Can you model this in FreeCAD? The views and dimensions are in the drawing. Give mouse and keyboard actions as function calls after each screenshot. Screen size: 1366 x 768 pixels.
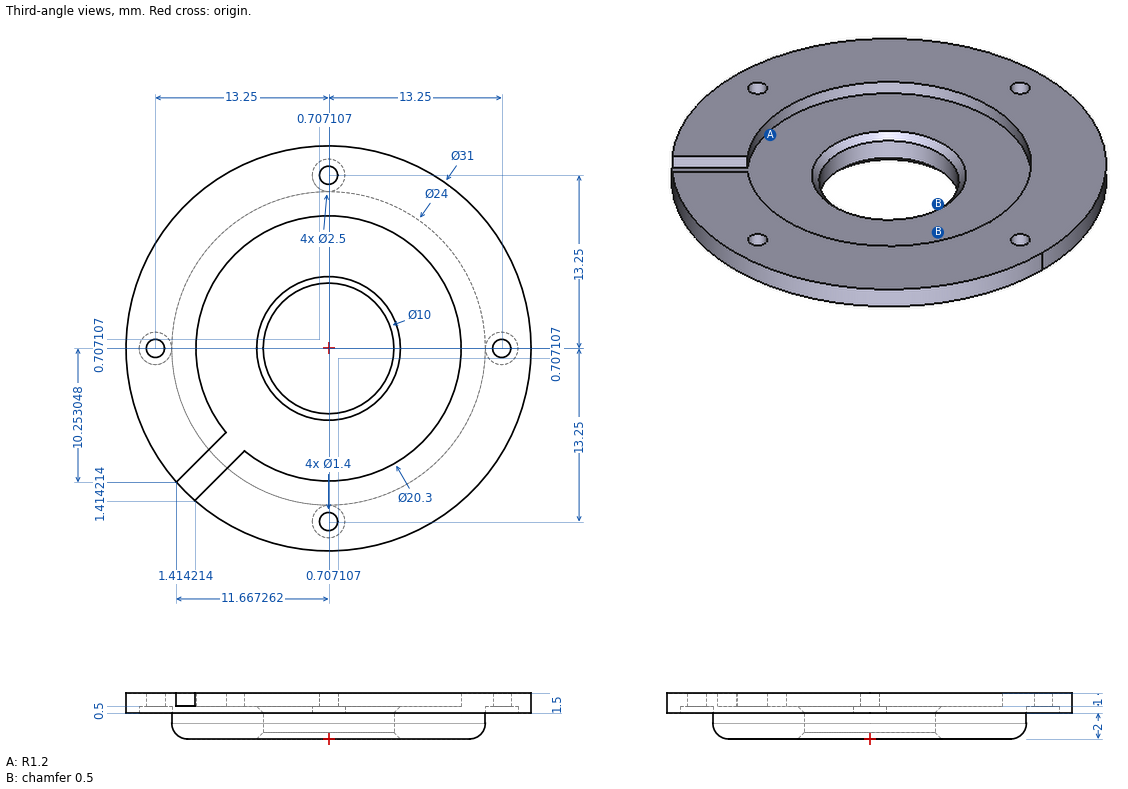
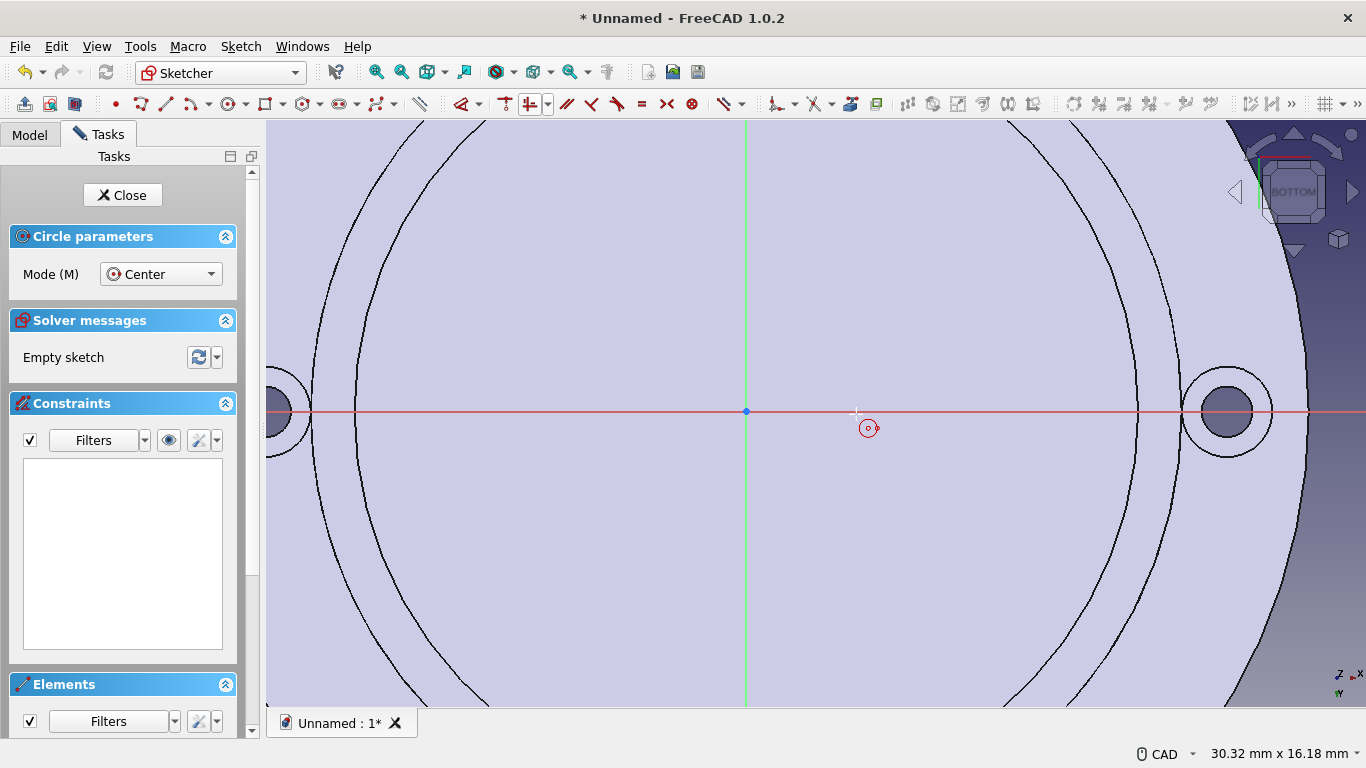
click(746, 412)
move(875, 284)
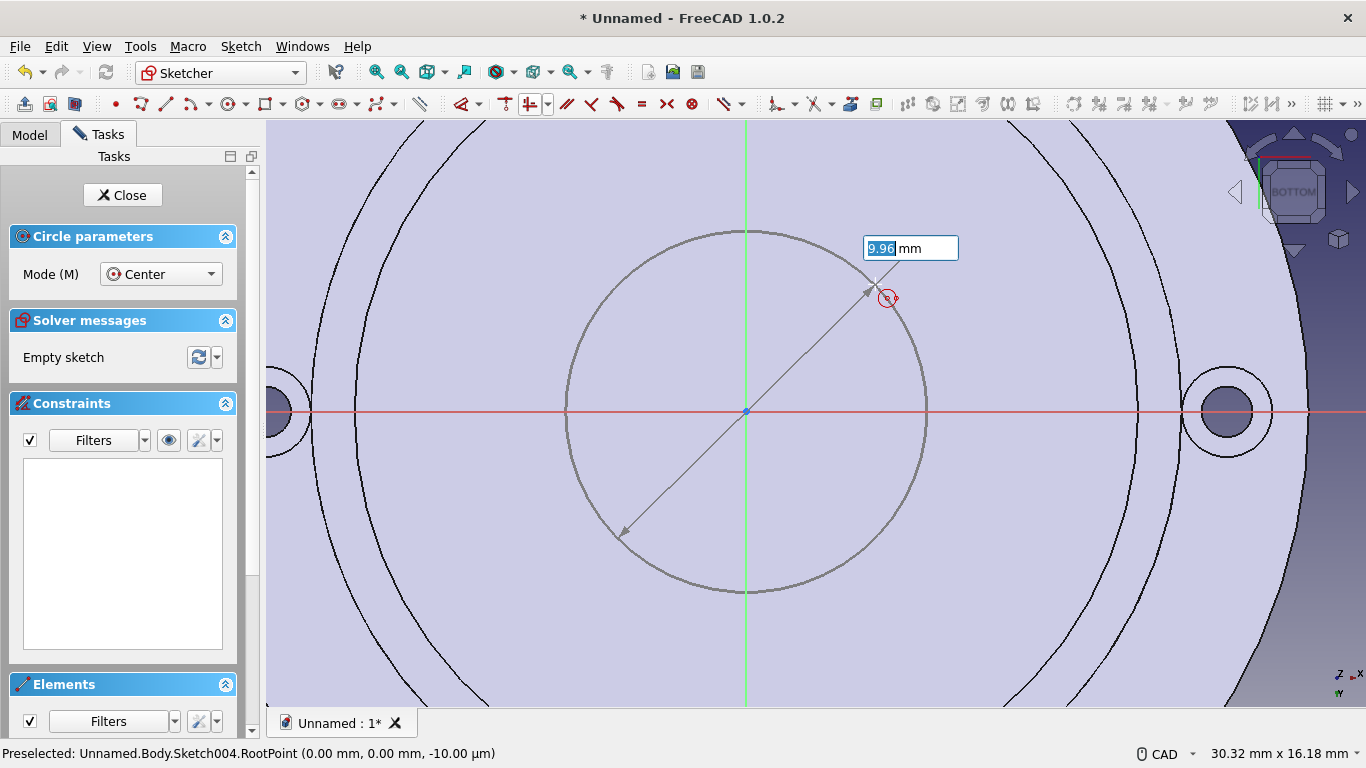
text(10)
key(Return)
key(Escape)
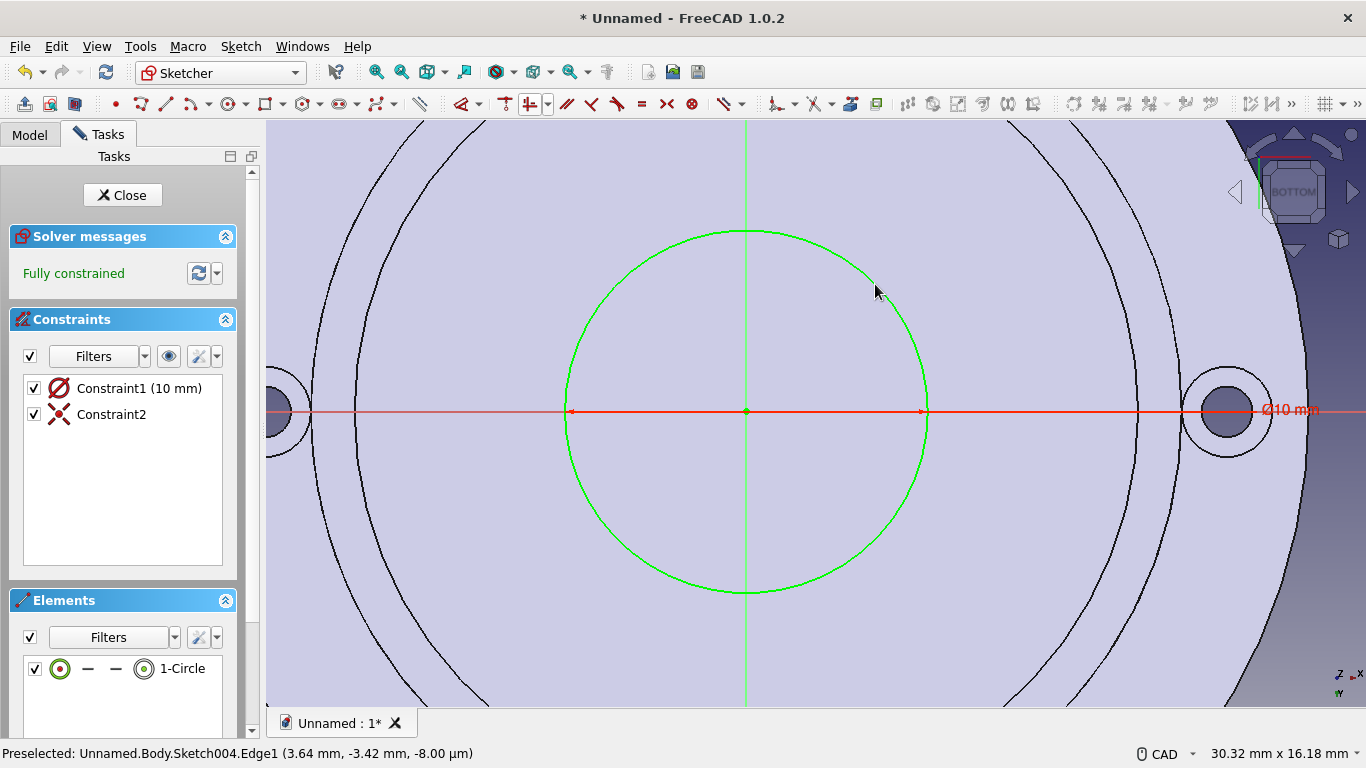
click(123, 195)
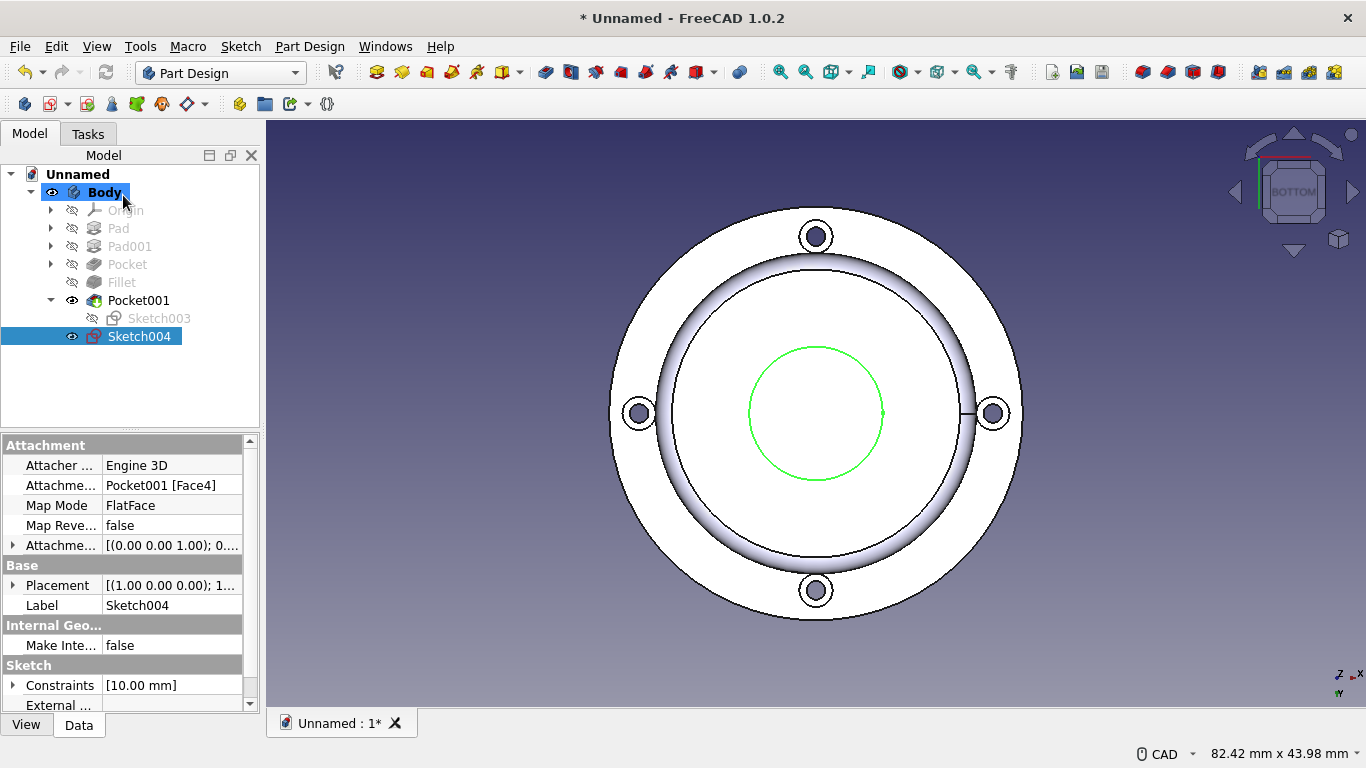
click(546, 72)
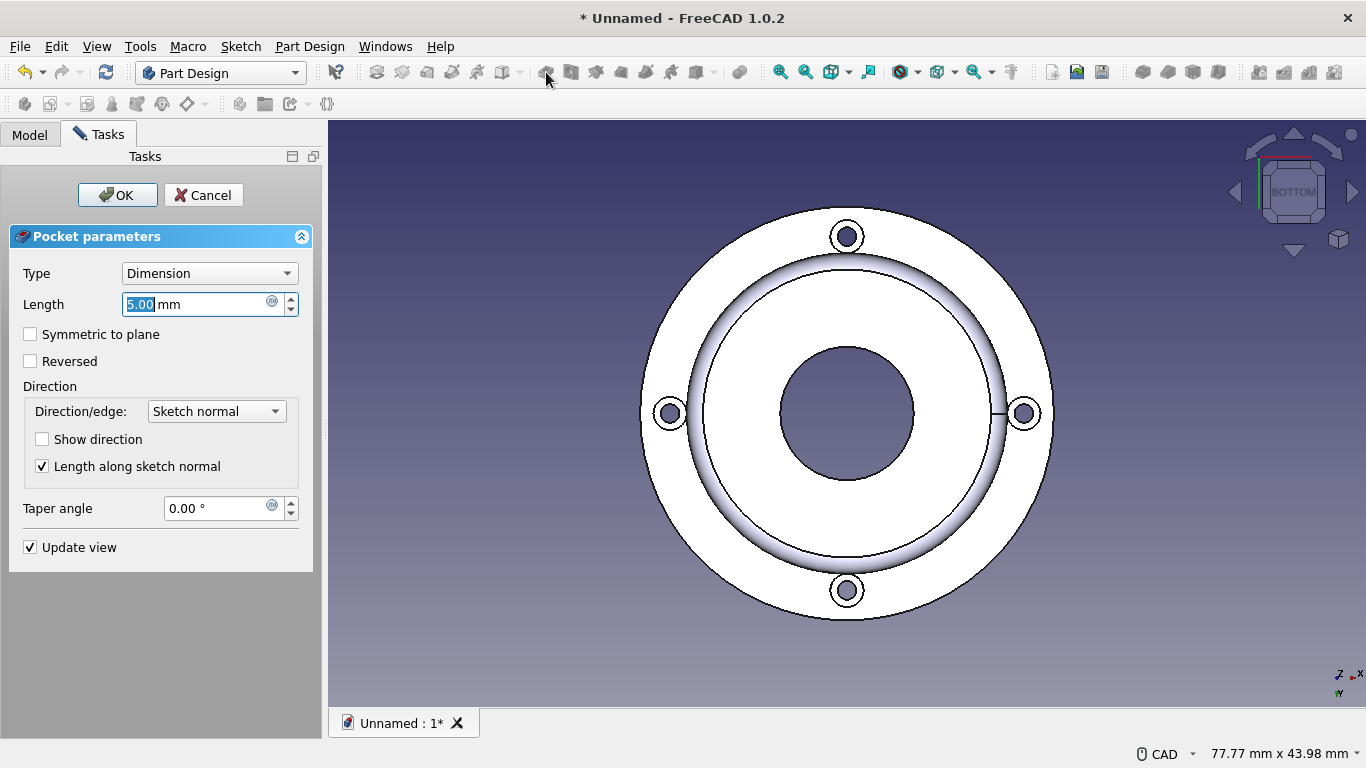
click(210, 274)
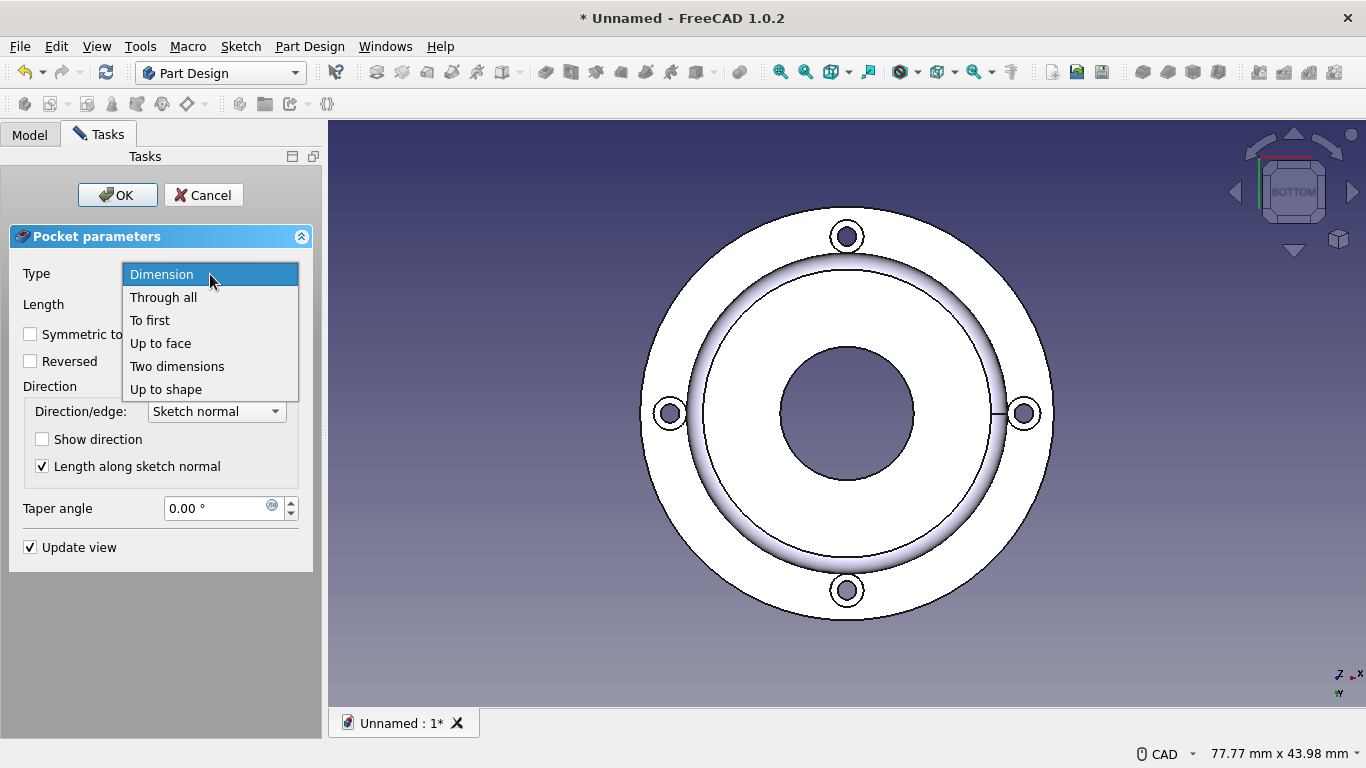
click(208, 298)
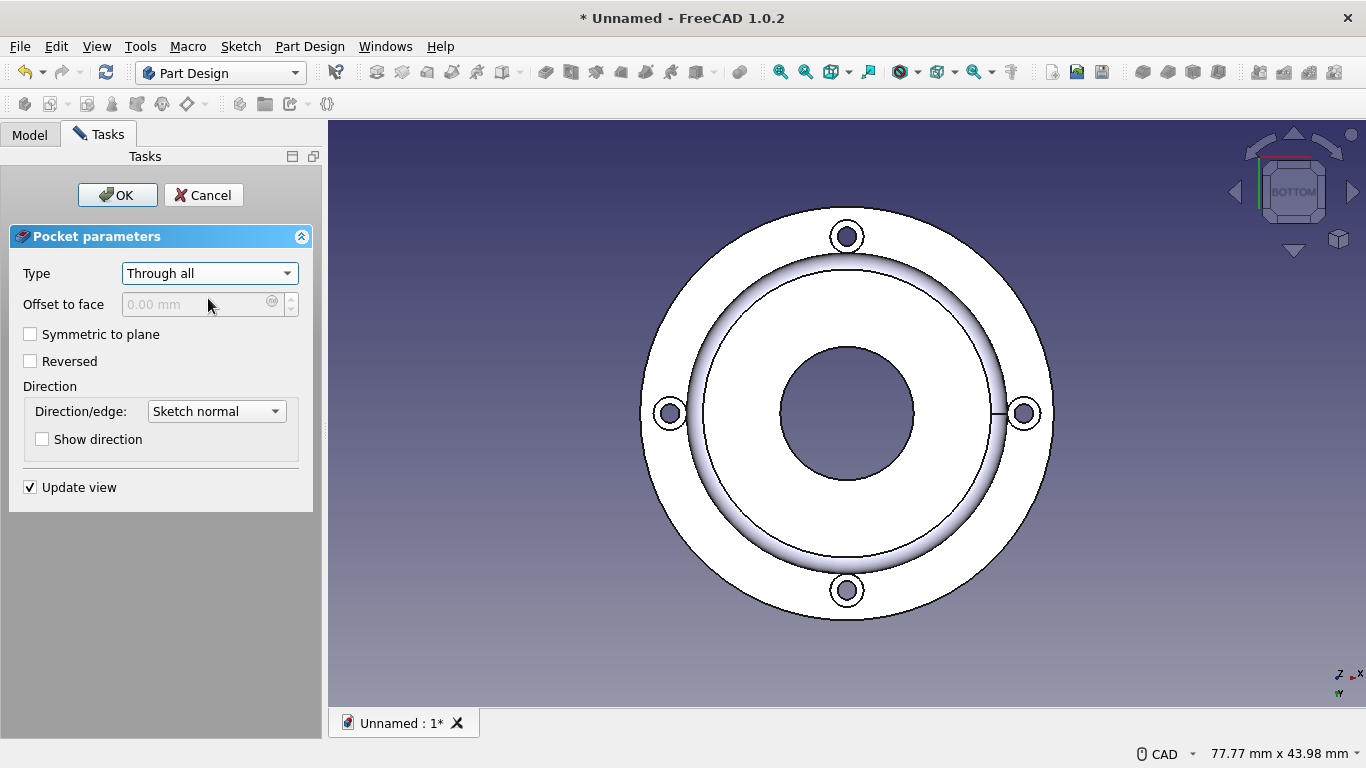
click(118, 195)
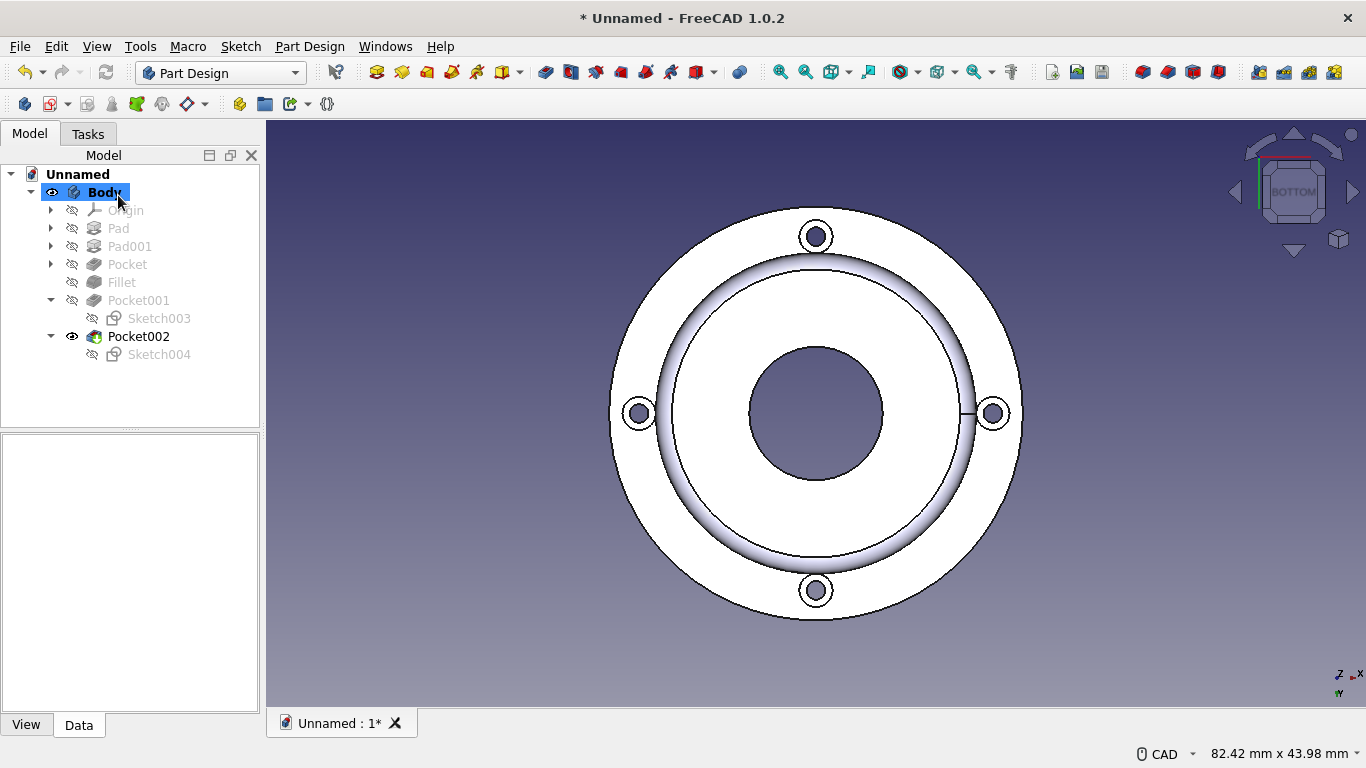
click(762, 373)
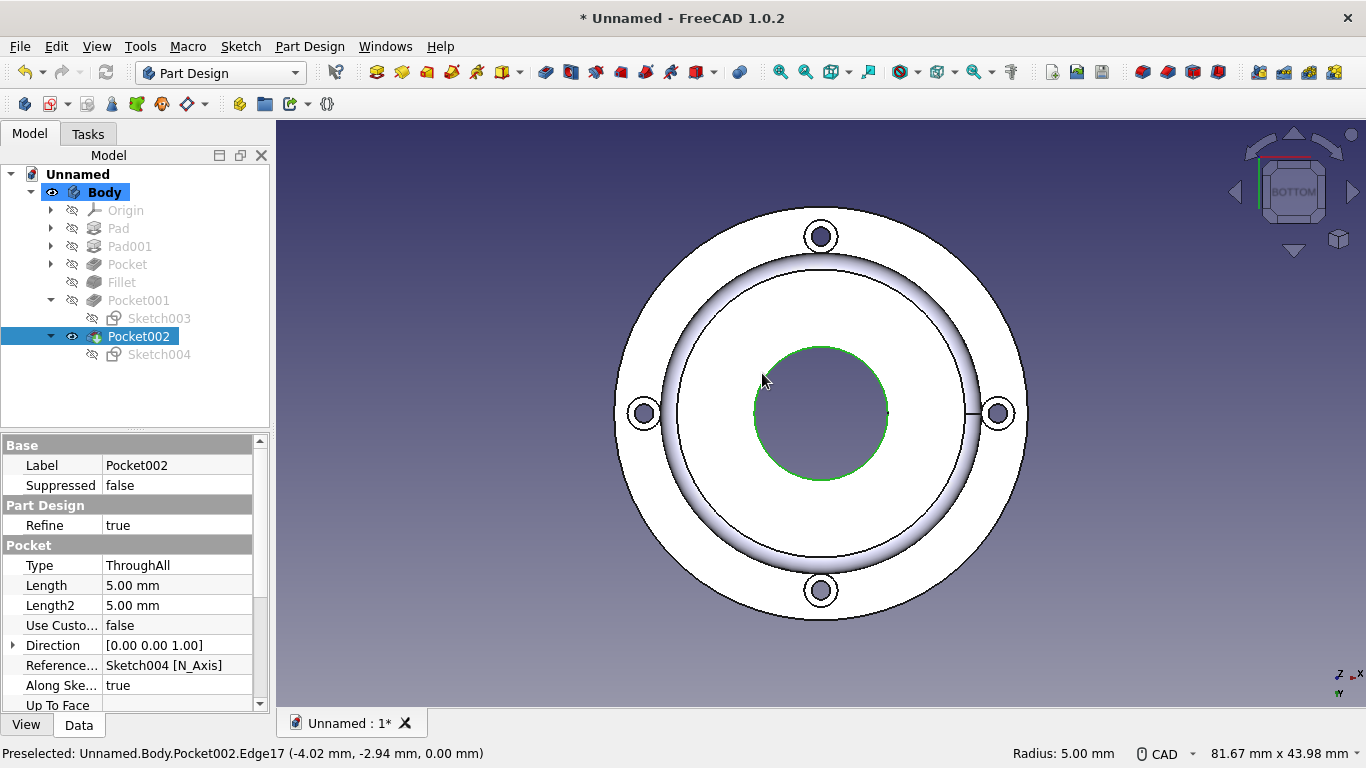
key(0)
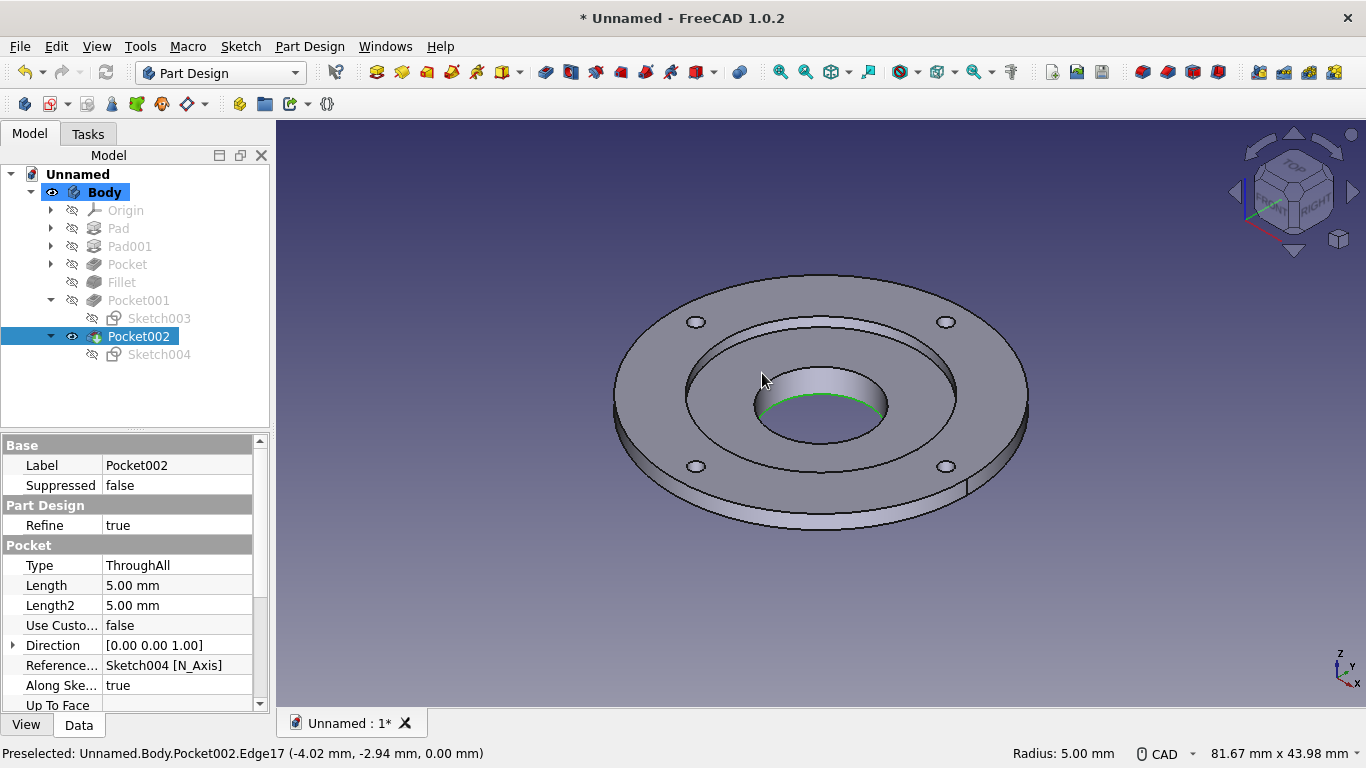
click(774, 377, ctrl)